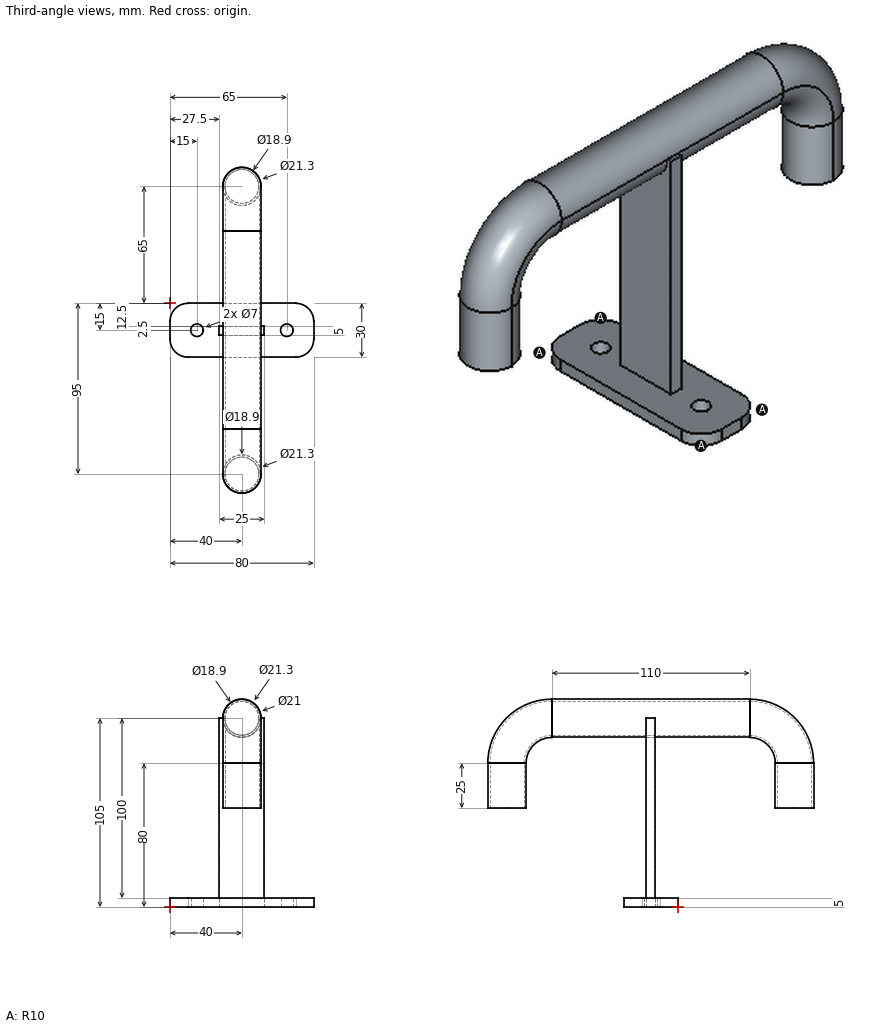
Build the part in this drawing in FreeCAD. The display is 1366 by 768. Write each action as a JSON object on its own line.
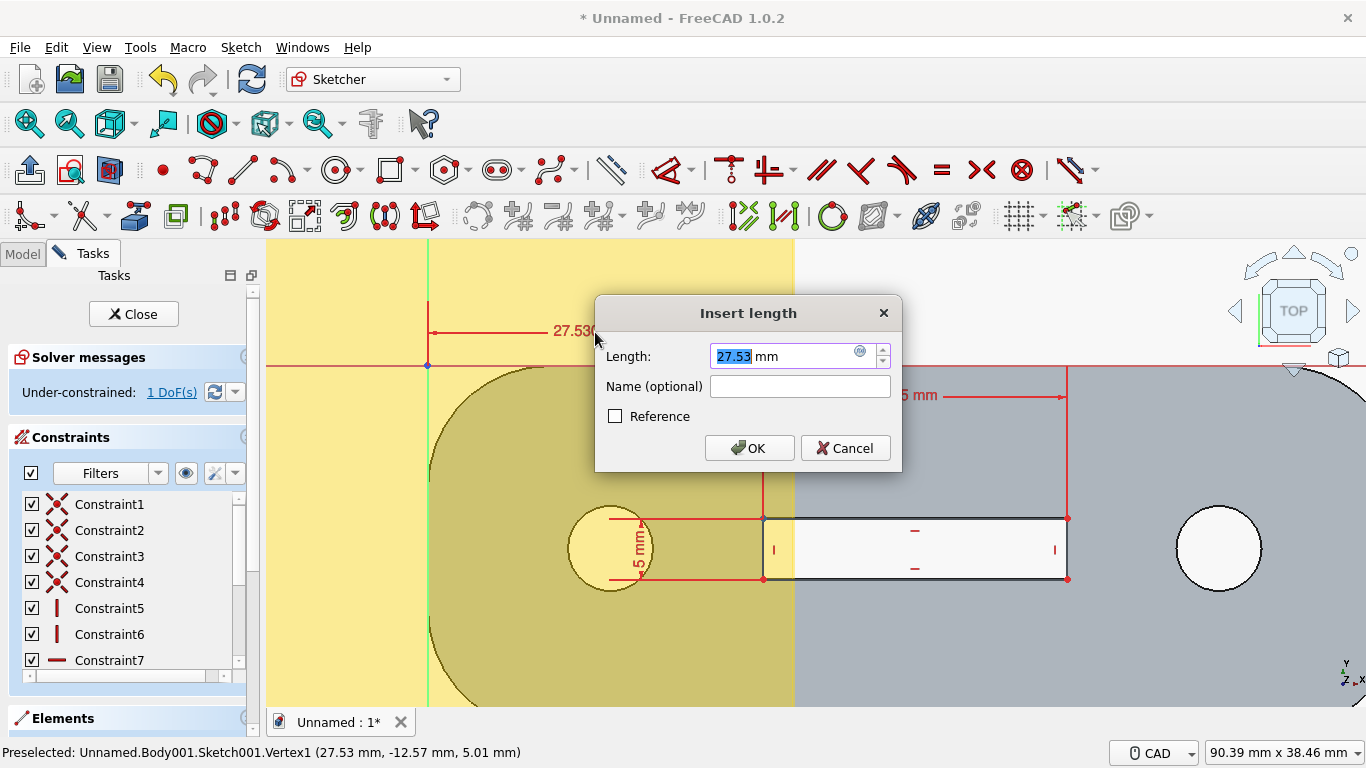
{"action": "type", "text": "27.5"}
{"action": "key", "text": "Return"}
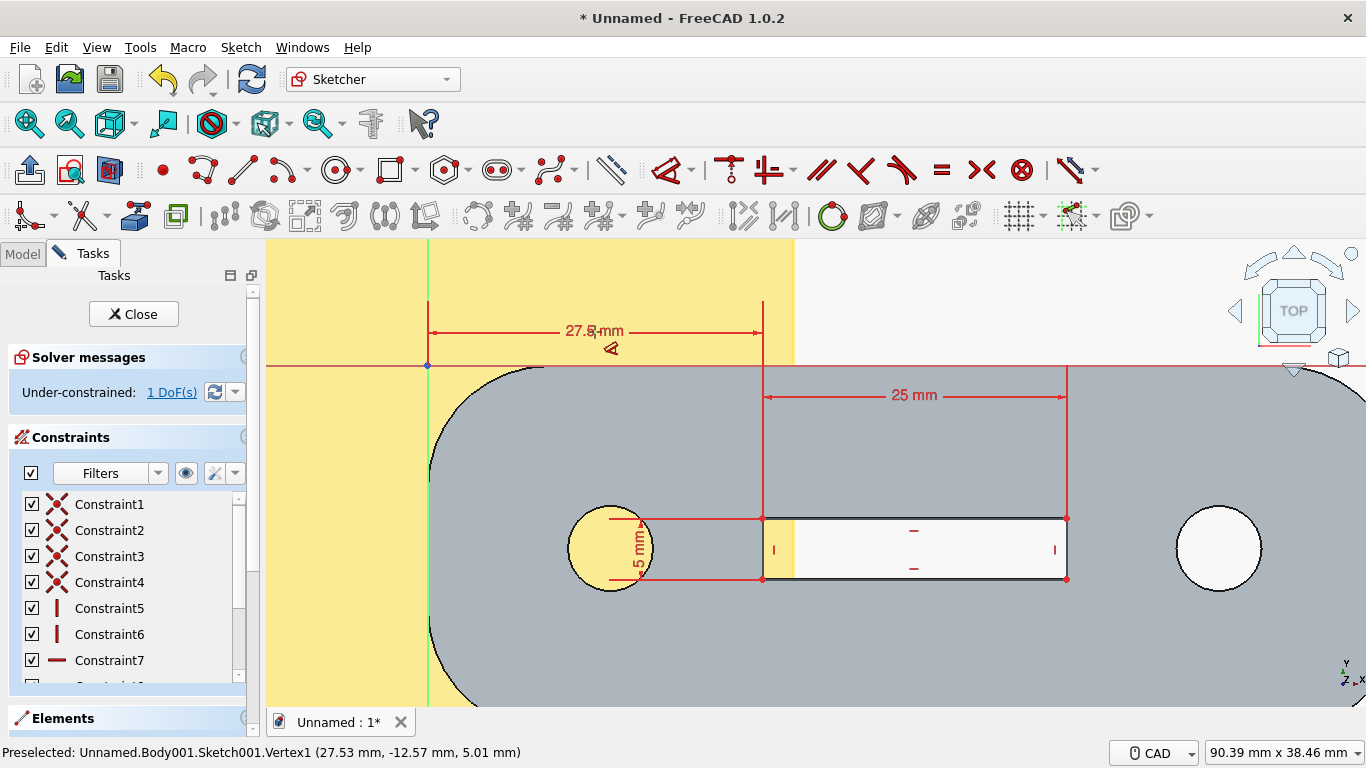
{"action": "left_click", "coordinate": [763, 519]}
{"action": "left_click", "coordinate": [394, 442]}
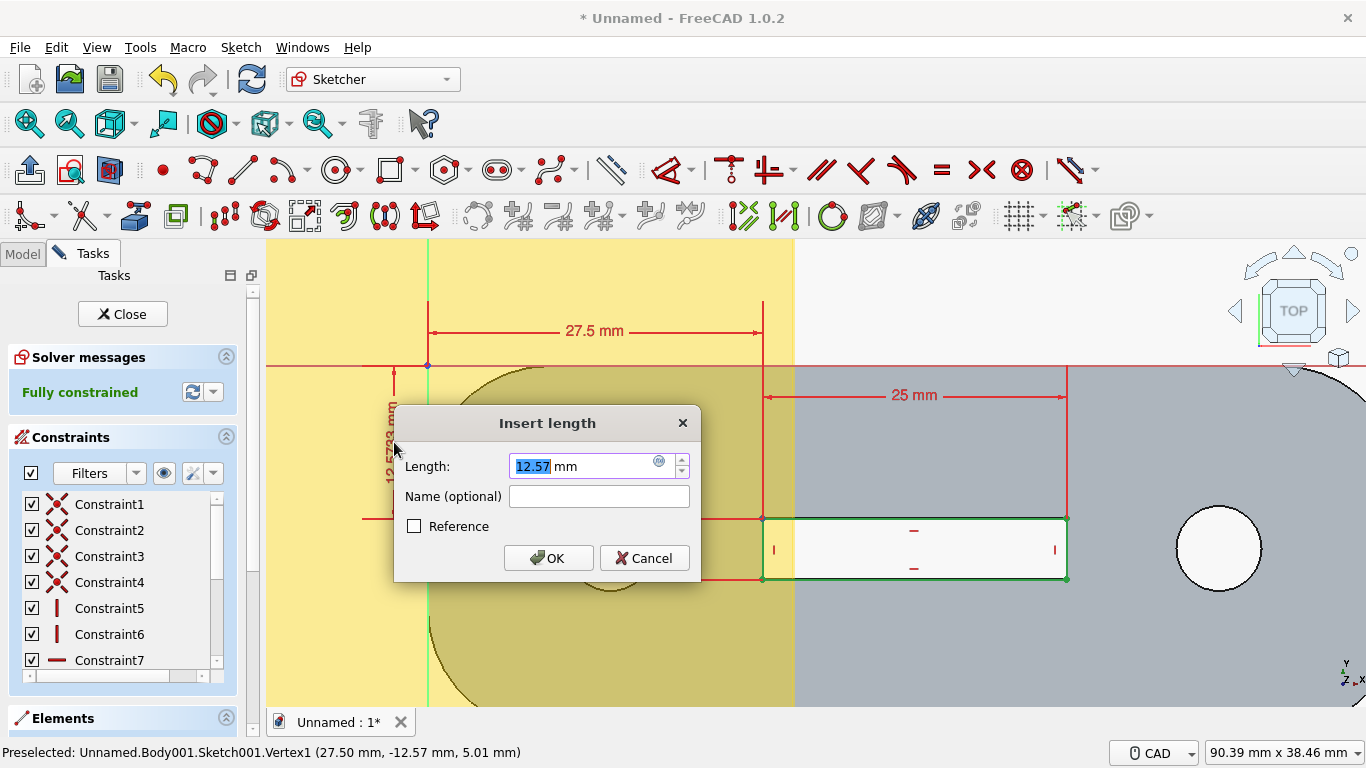
{"action": "type", "text": "12.5"}
{"action": "key", "text": "Return"}
{"action": "key", "text": "Escape"}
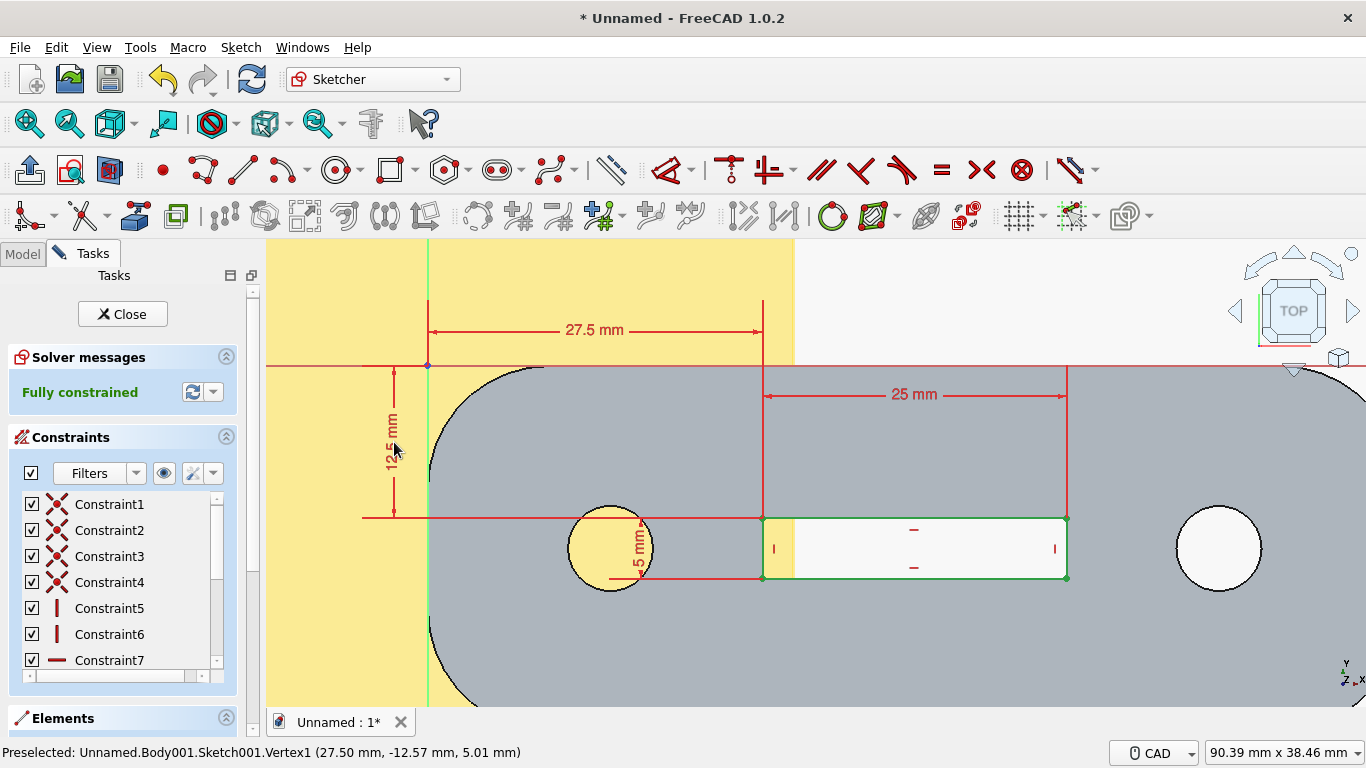
{"action": "left_click", "coordinate": [123, 314]}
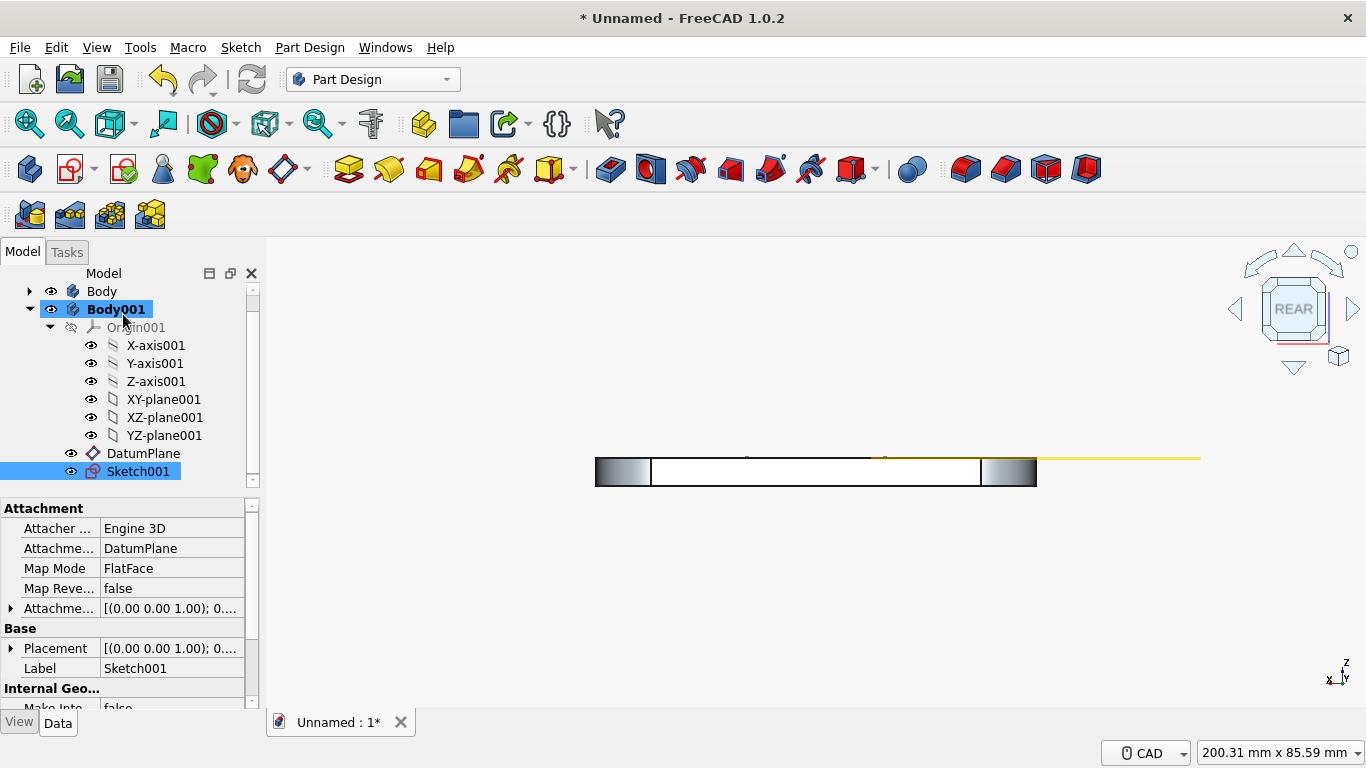
{"action": "left_click", "coordinate": [350, 170]}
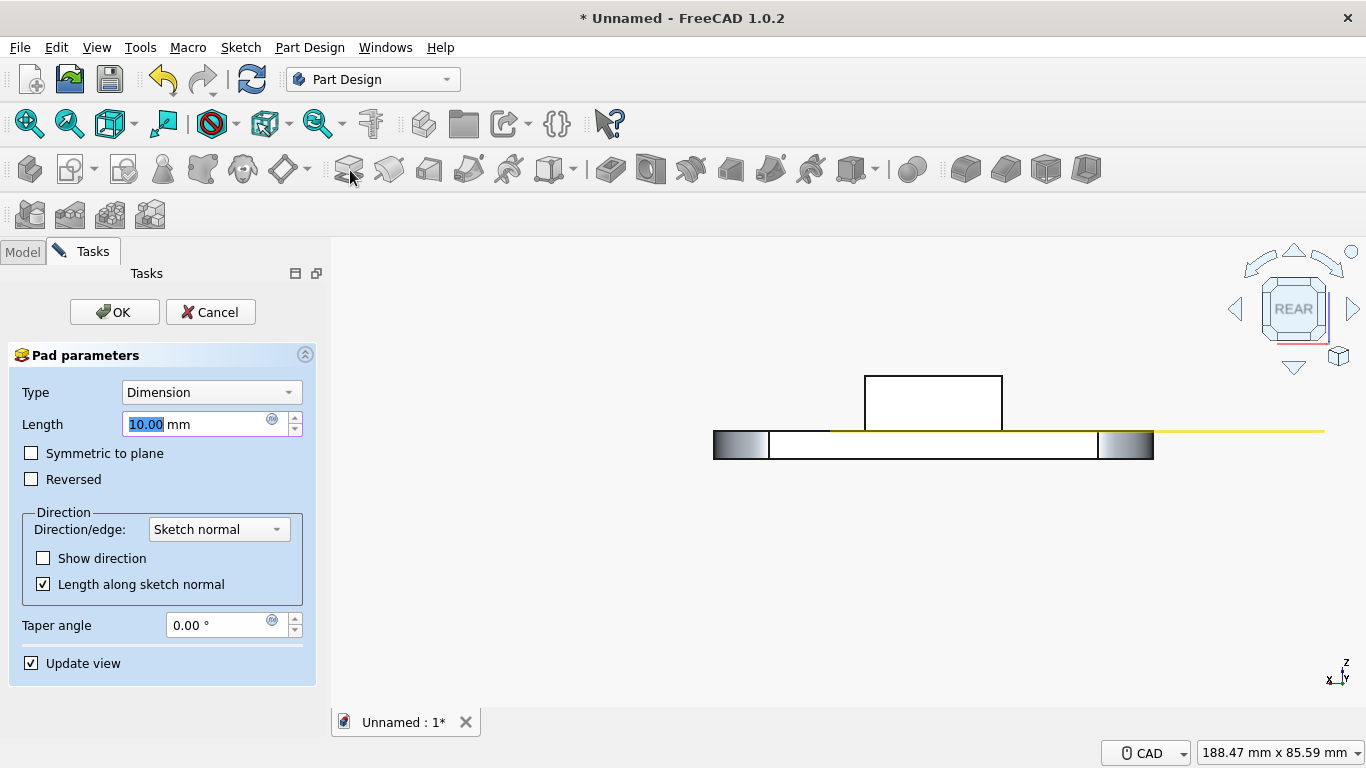
{"action": "type", "text": "100"}
{"action": "key", "text": "Tab"}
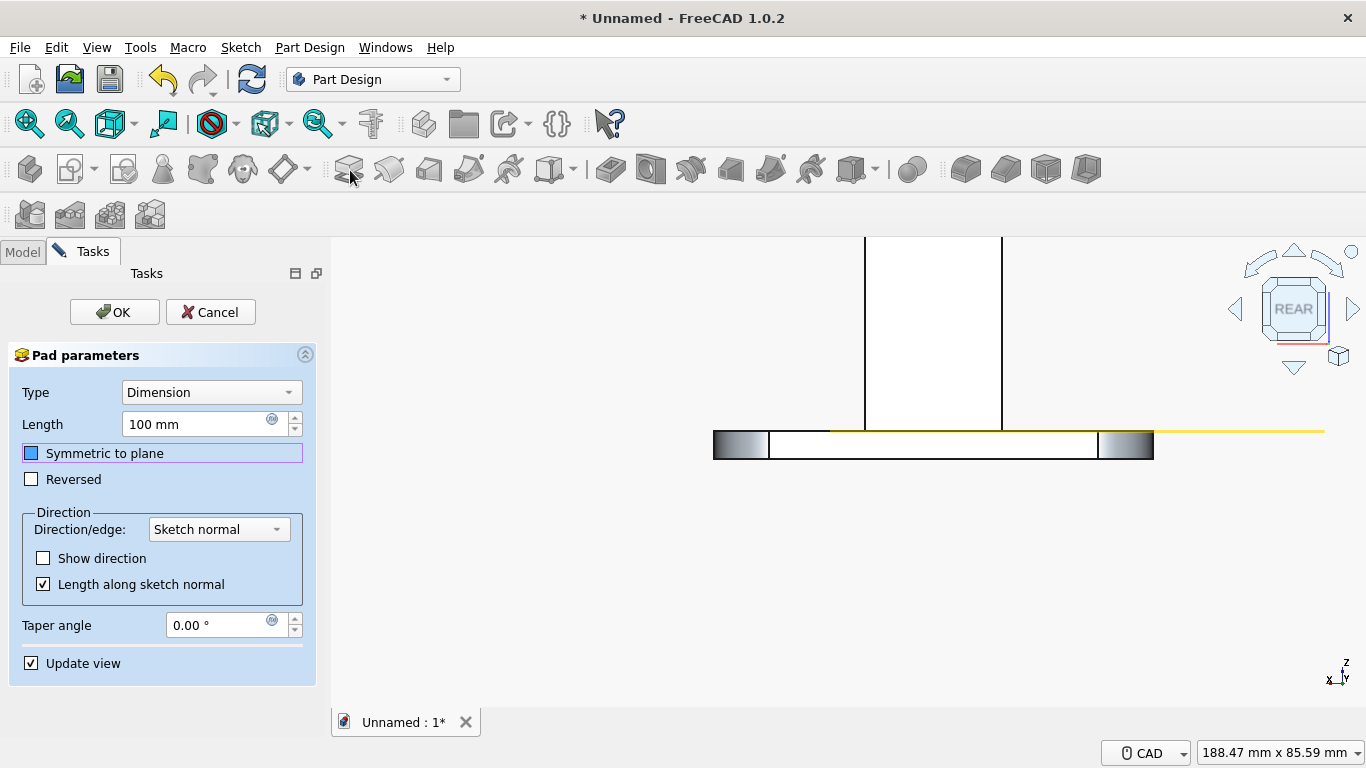
{"action": "left_click", "coordinate": [115, 312]}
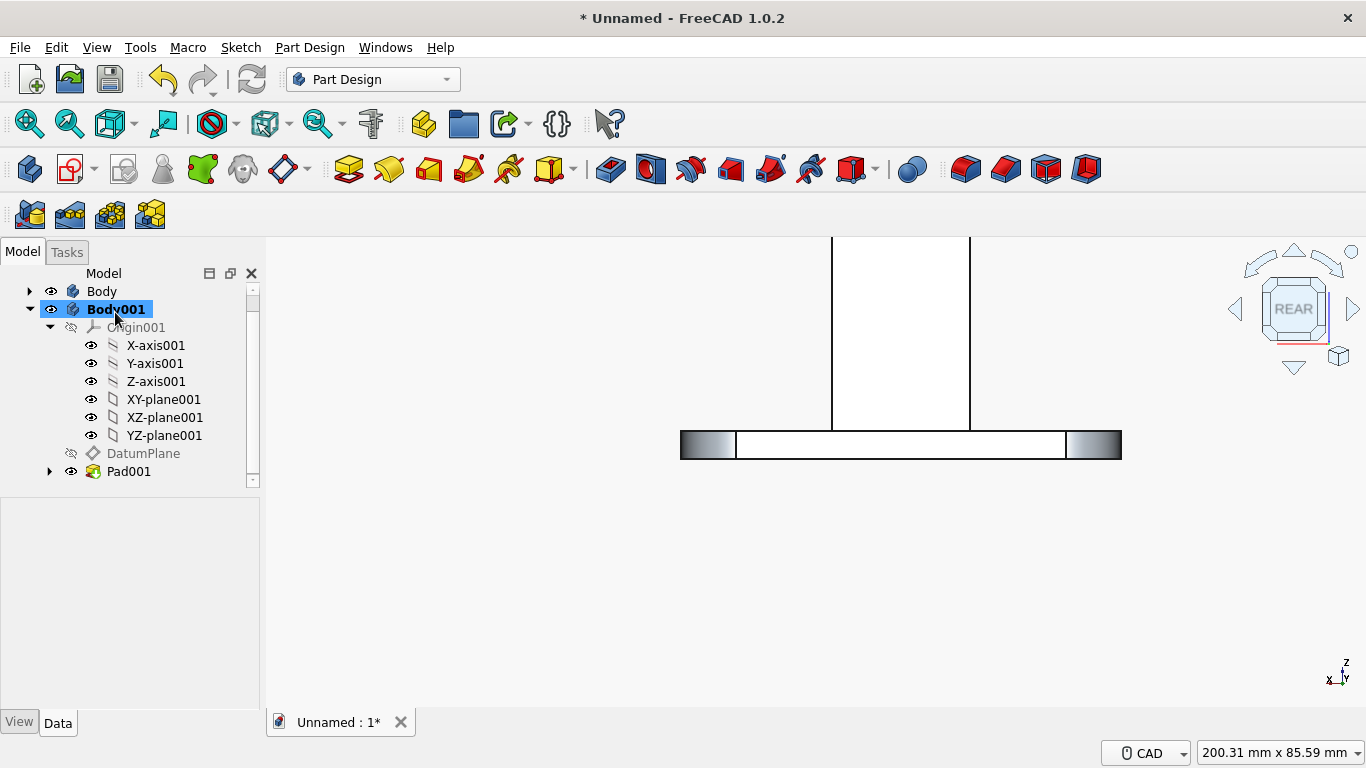
{"action": "left_click", "coordinate": [30, 124]}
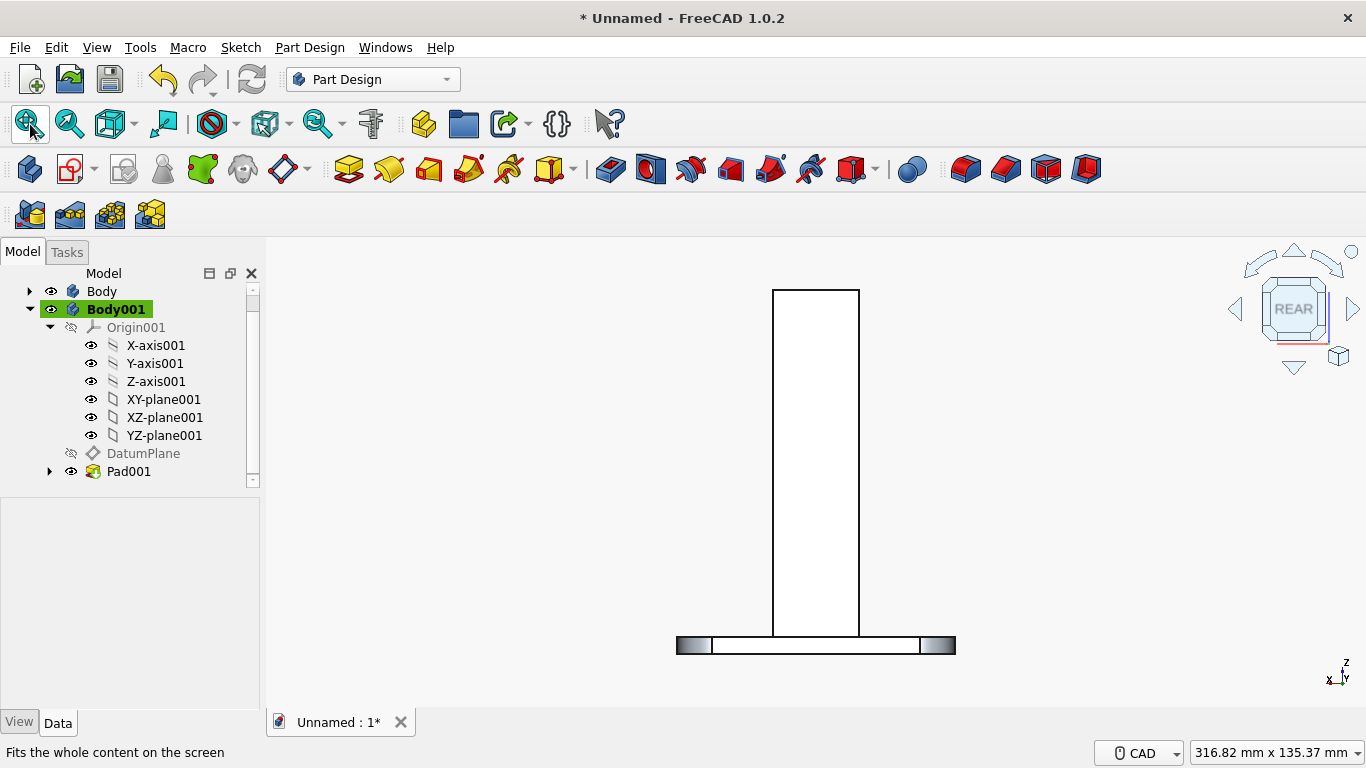
{"action": "key", "text": "0"}